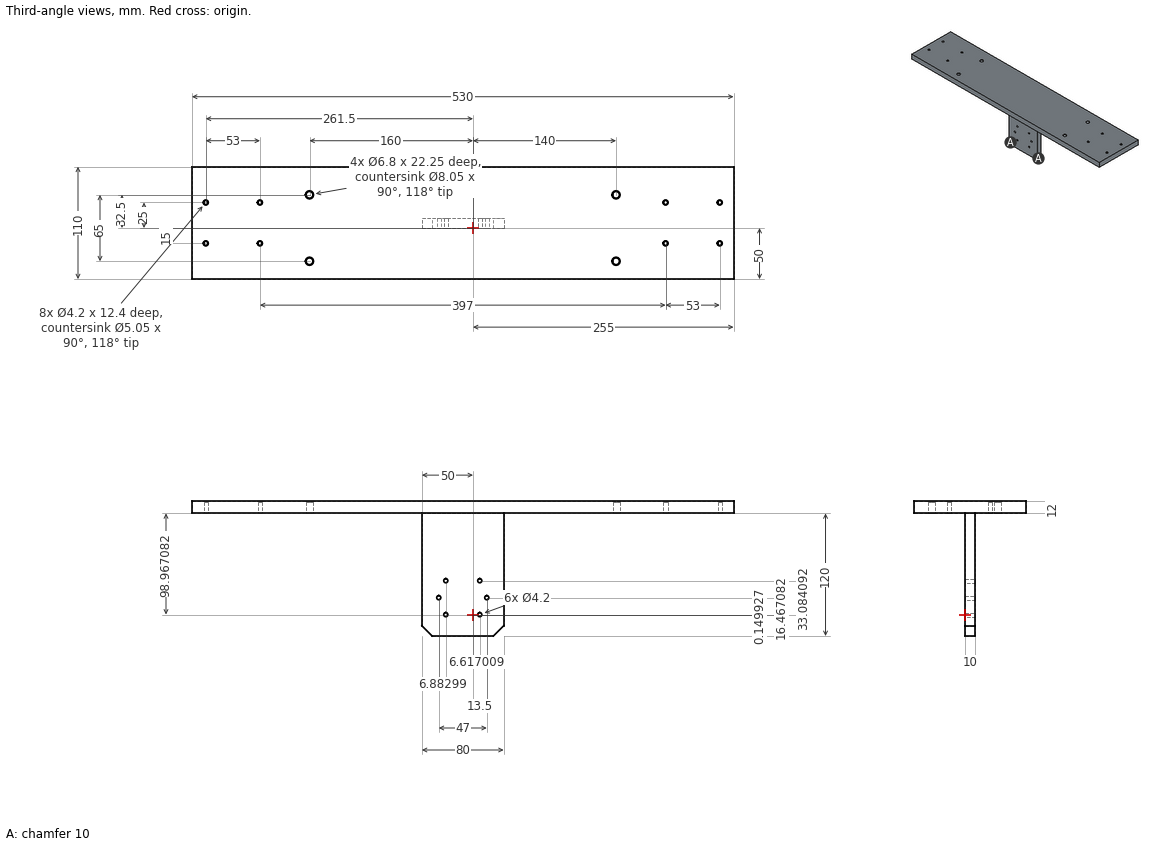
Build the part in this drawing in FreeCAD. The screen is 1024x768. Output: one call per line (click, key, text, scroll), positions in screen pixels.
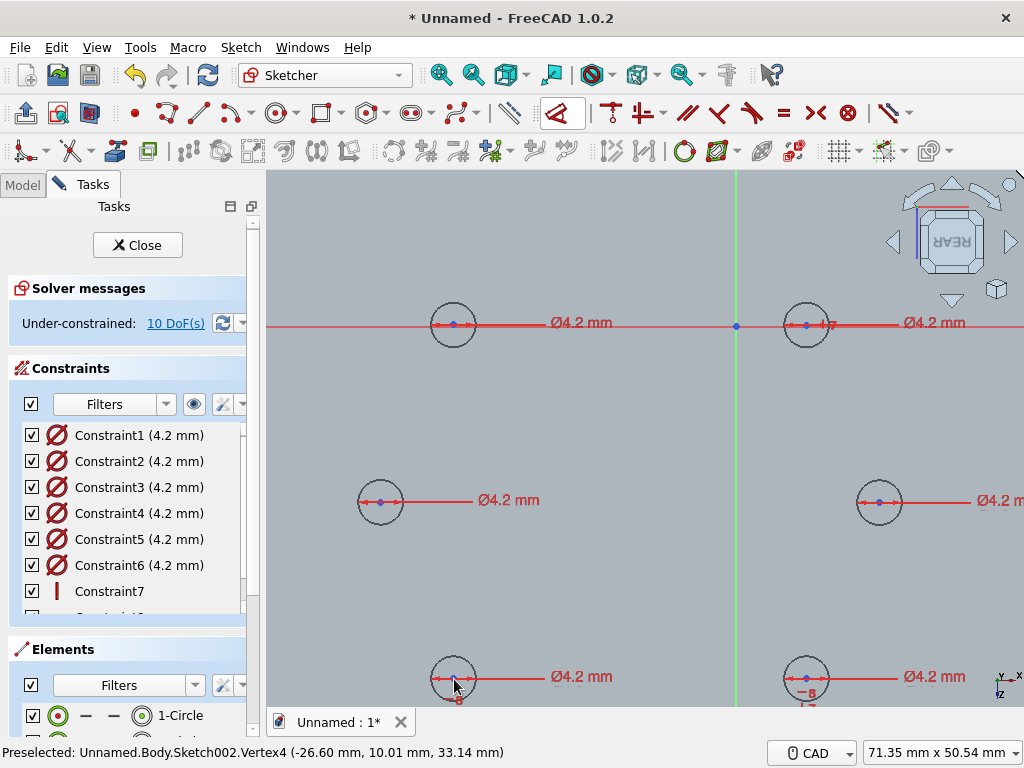
scroll(468, 310, down, 2)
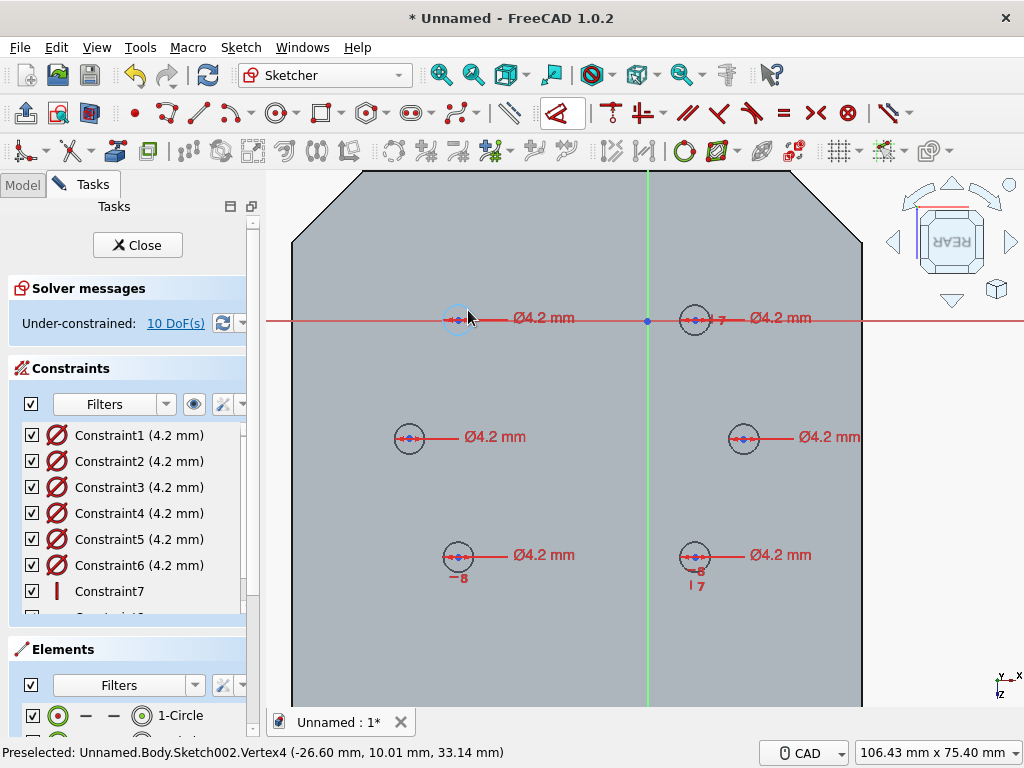
click(744, 439)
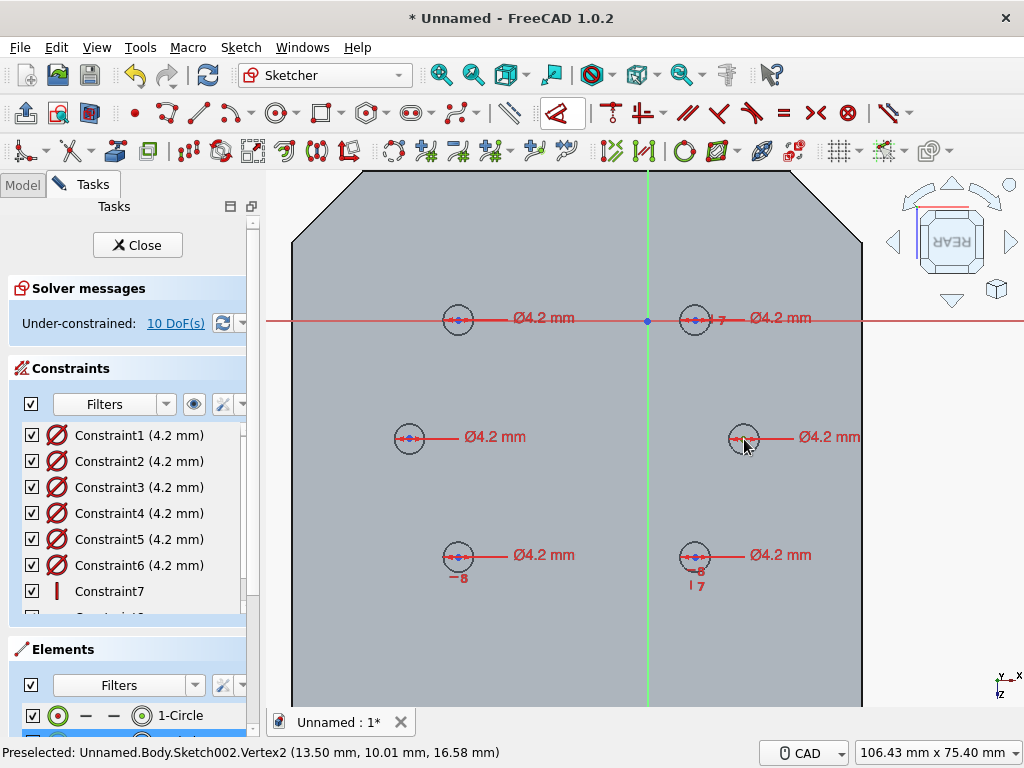
click(410, 439)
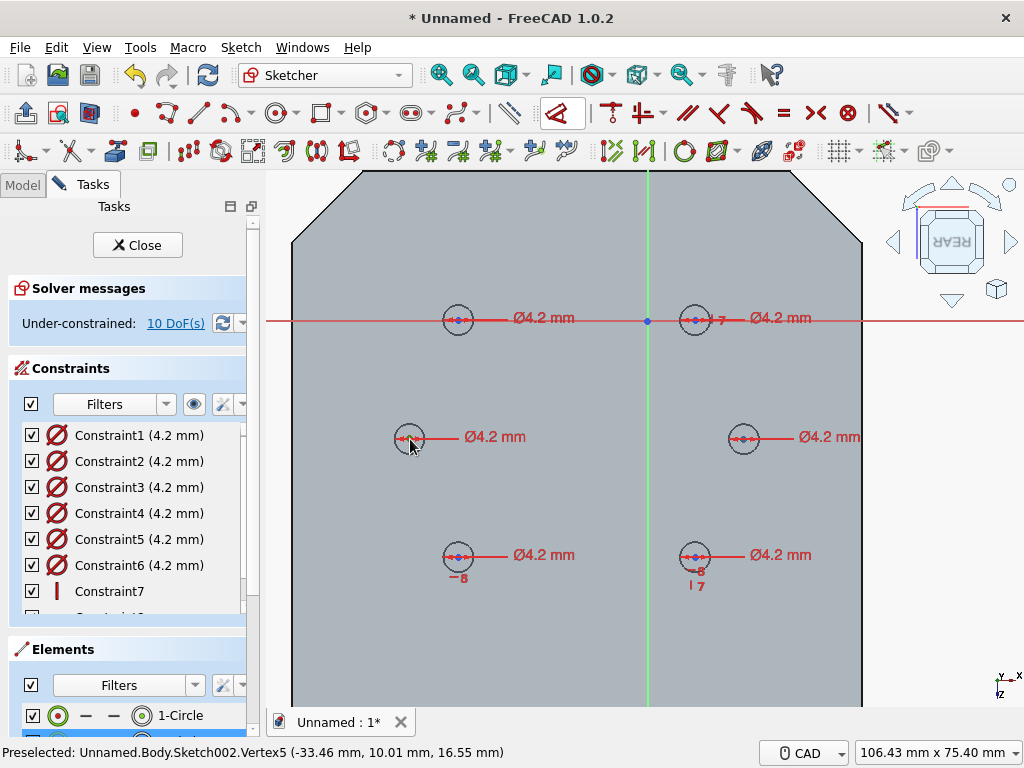
key(h)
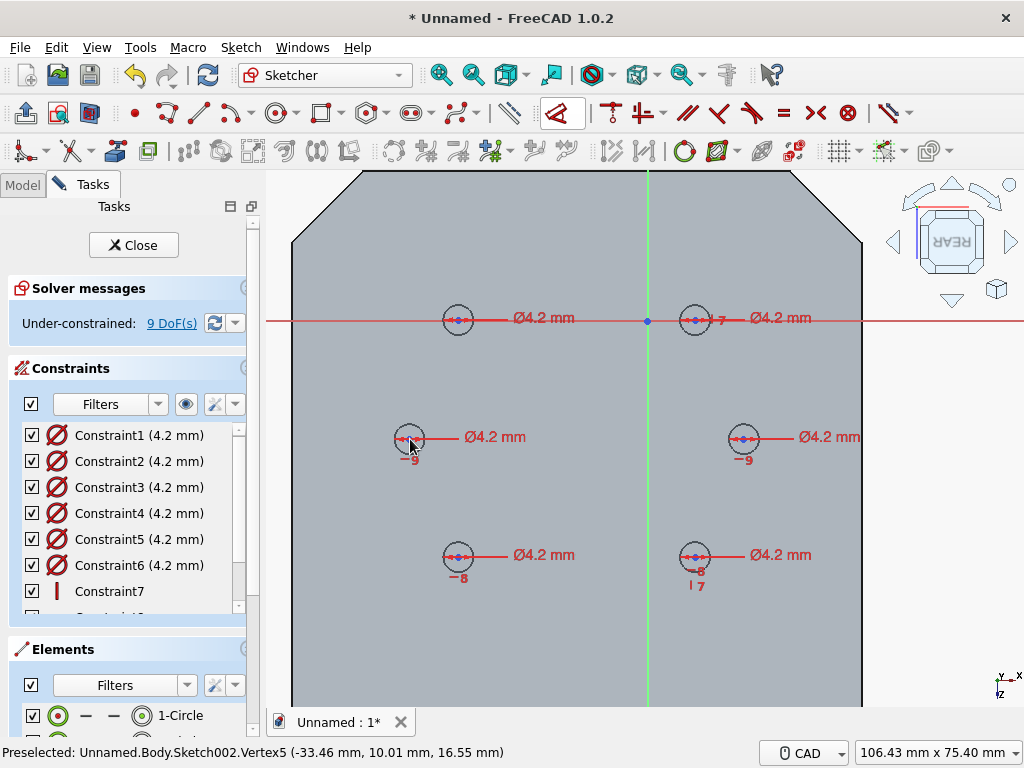
click(458, 557)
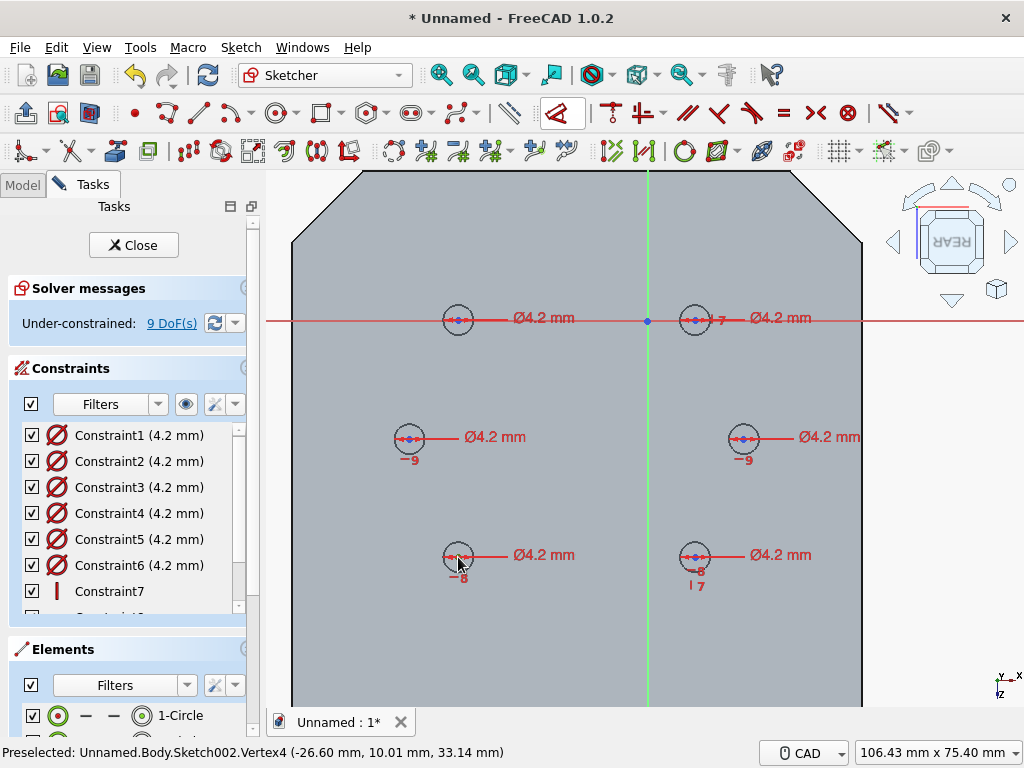
click(458, 320)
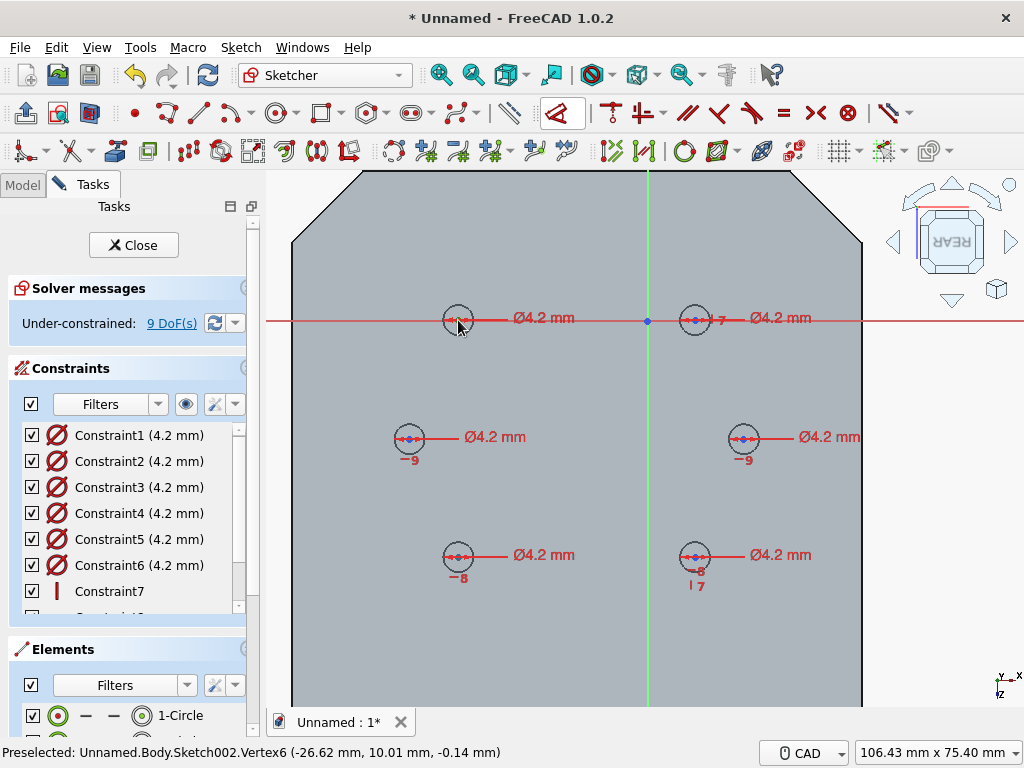
key(v)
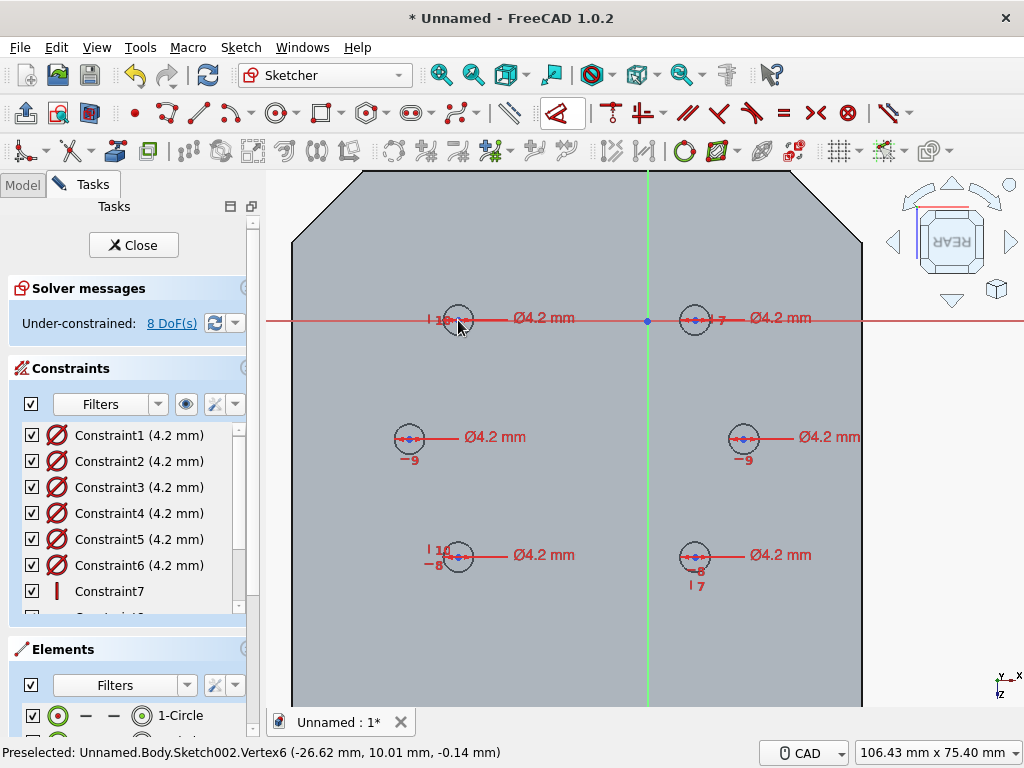
click(695, 320)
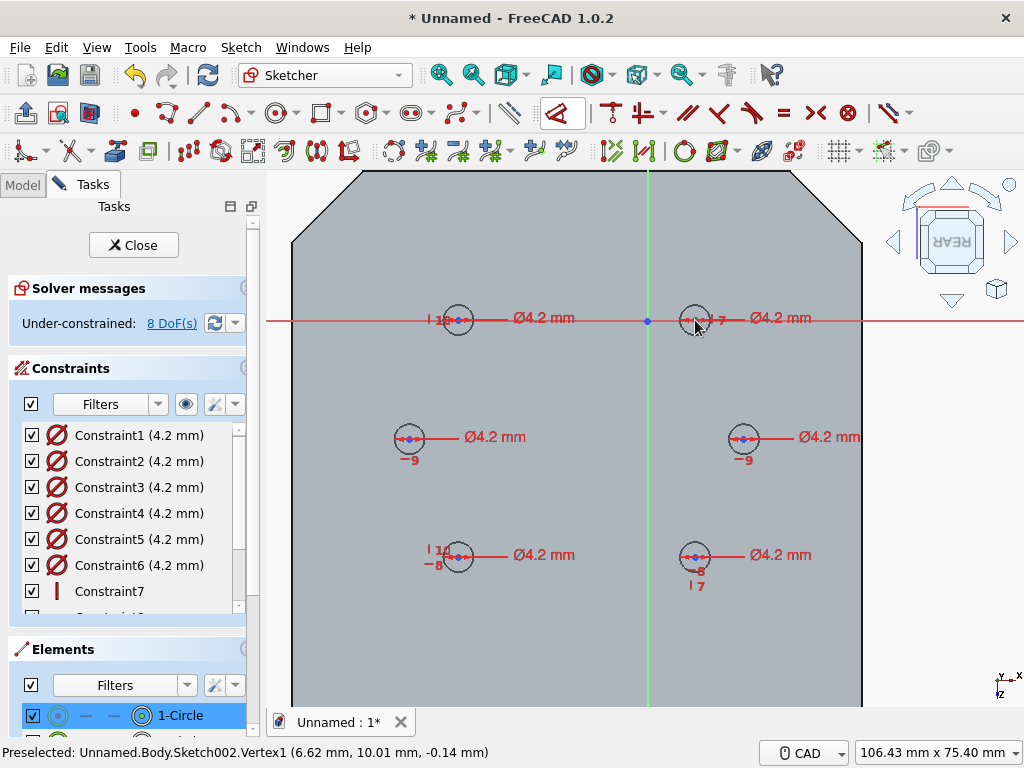
click(458, 320)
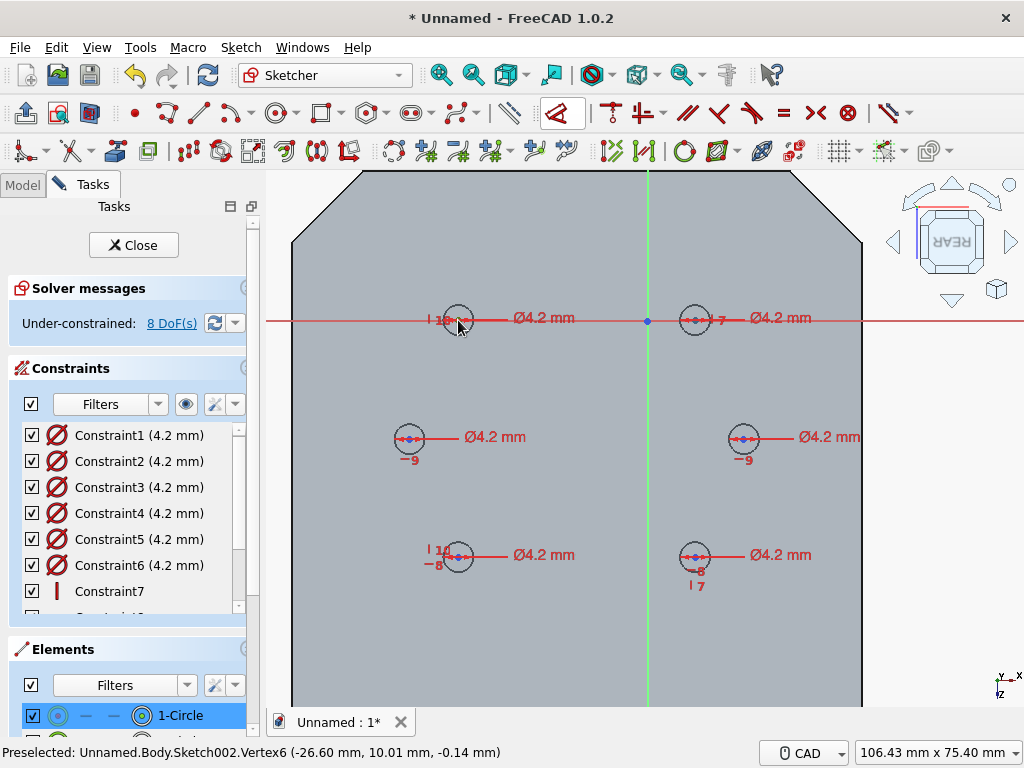
key(h)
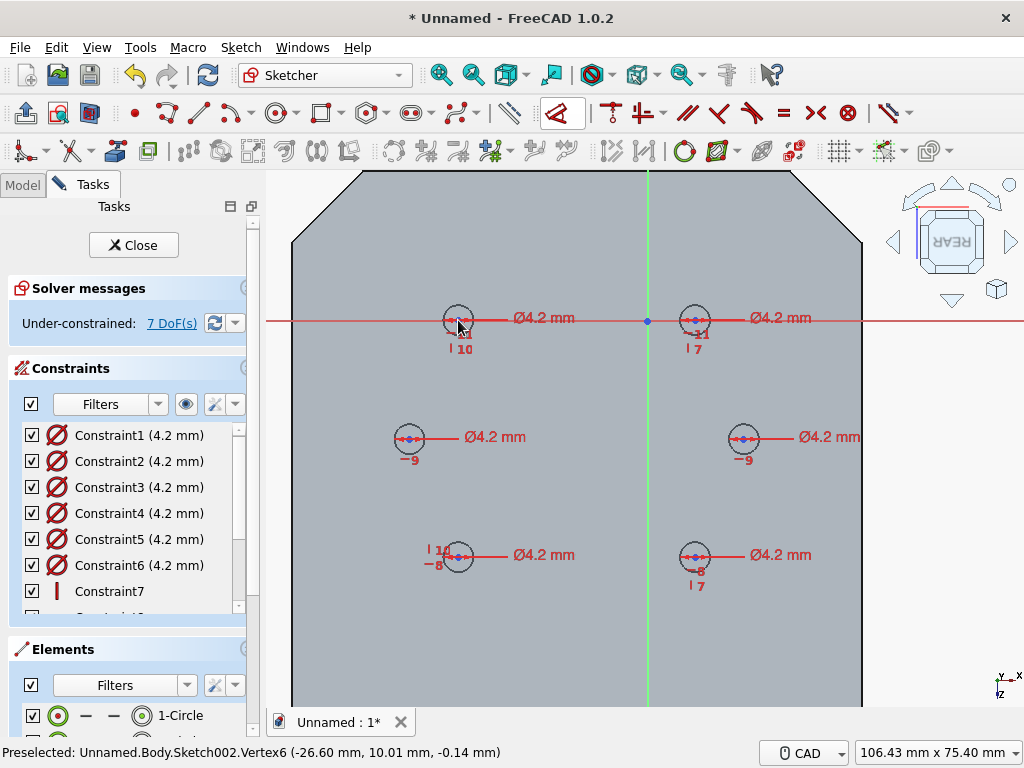
click(744, 439)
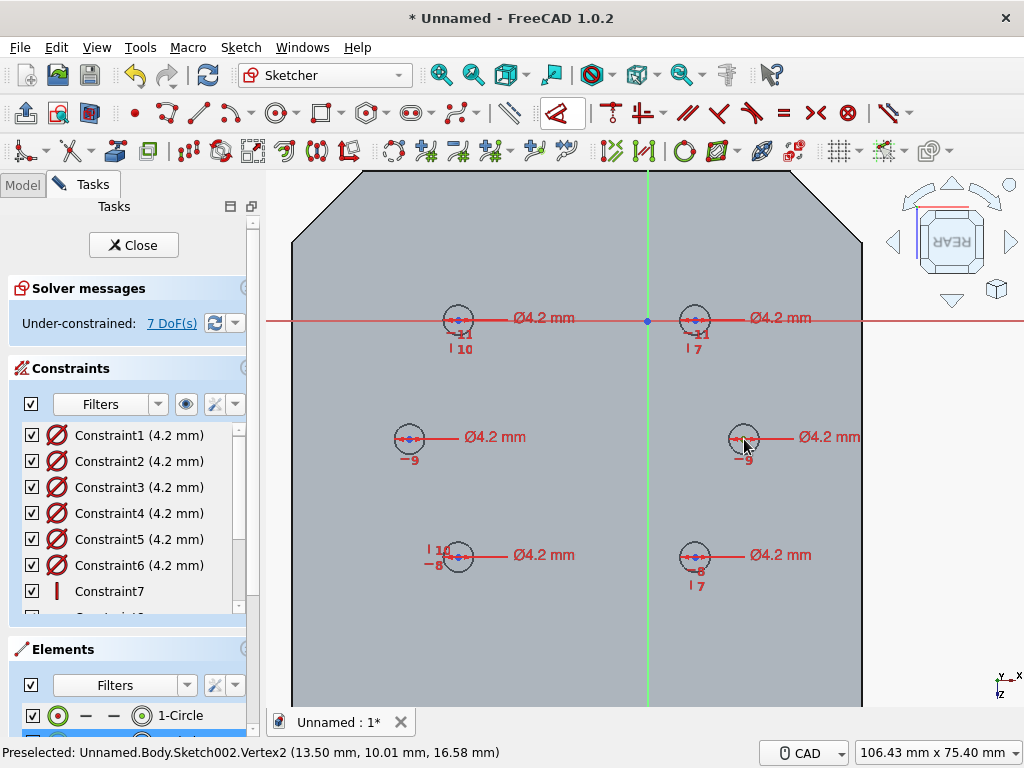
click(410, 439)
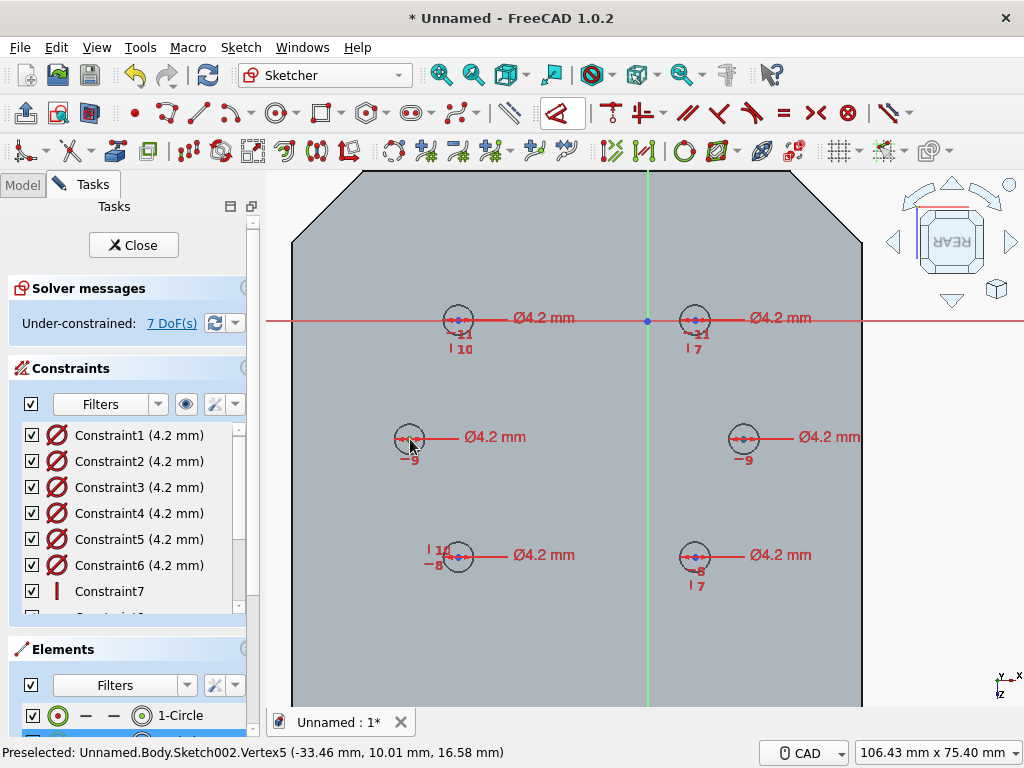
key(l)